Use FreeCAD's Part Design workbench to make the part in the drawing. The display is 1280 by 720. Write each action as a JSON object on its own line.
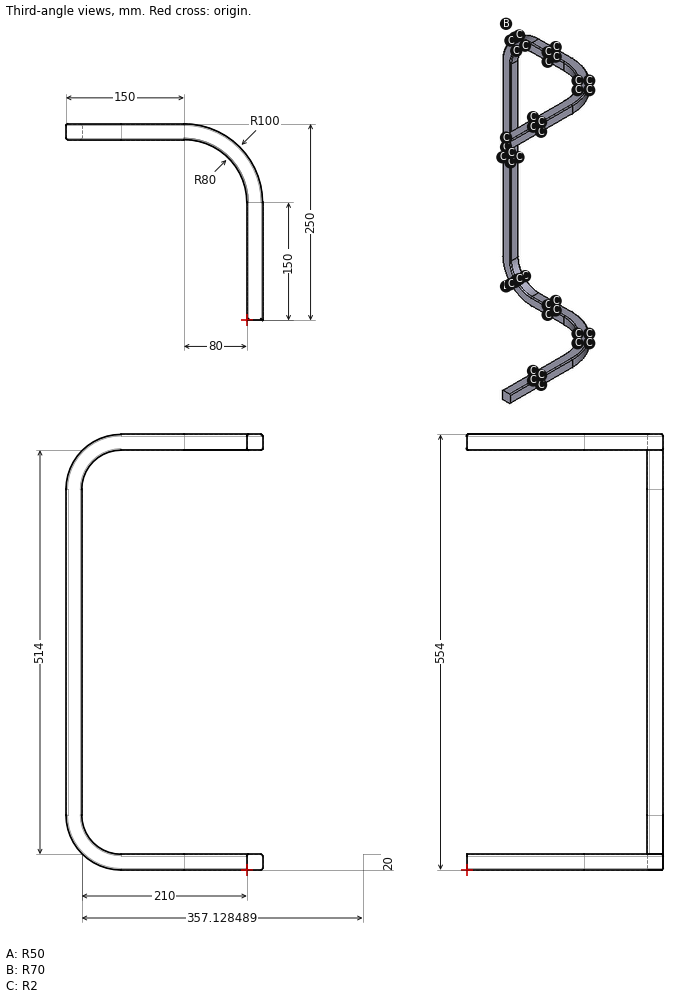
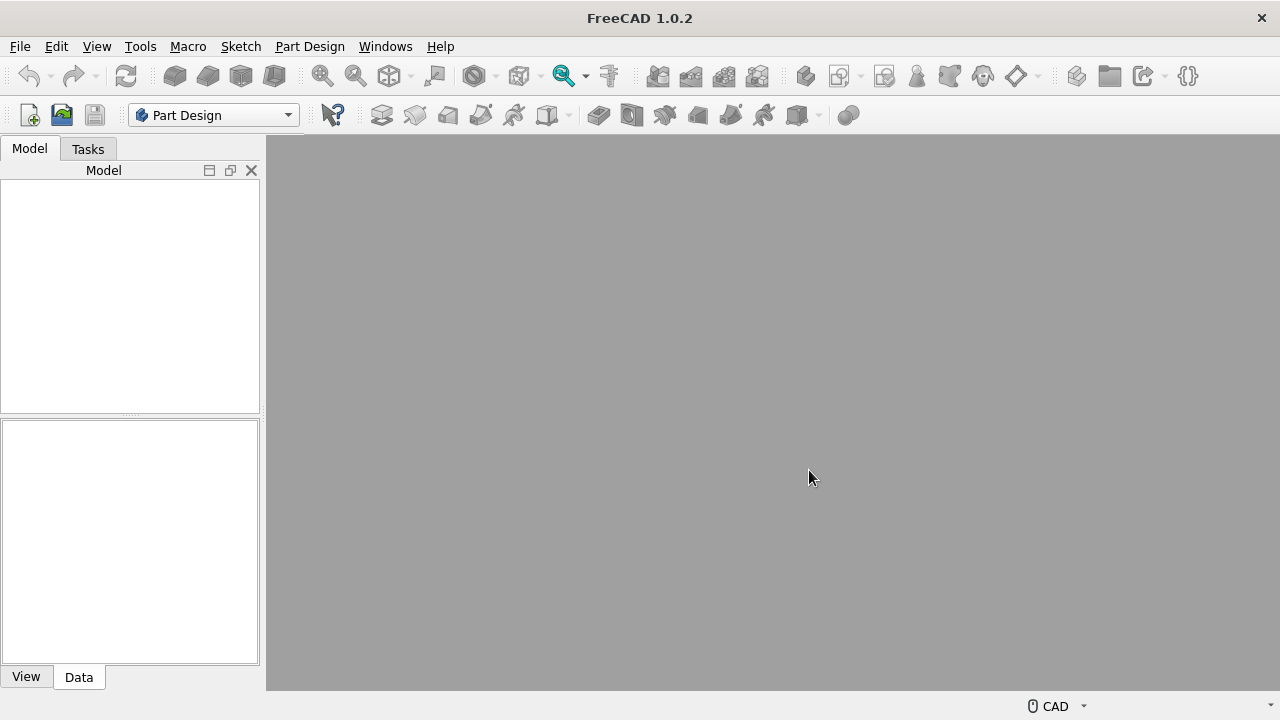
{"action": "left_click", "coordinate": [29, 116]}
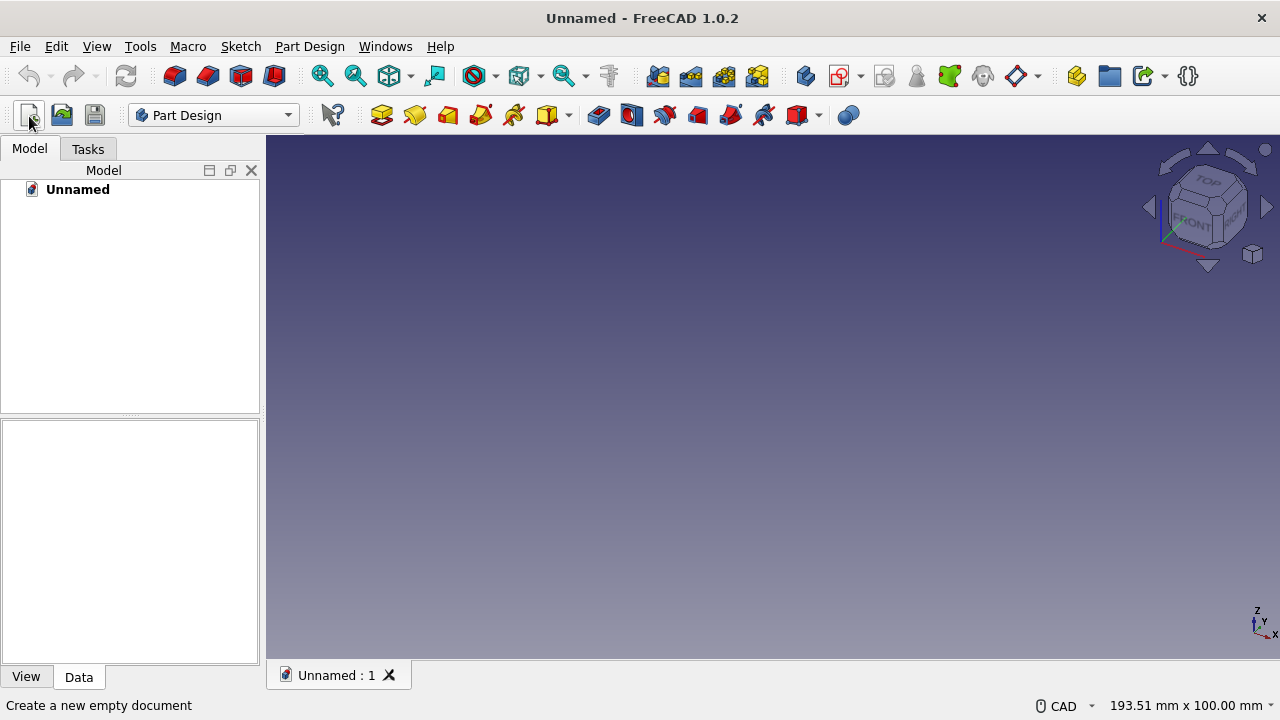
{"action": "left_click", "coordinate": [838, 76]}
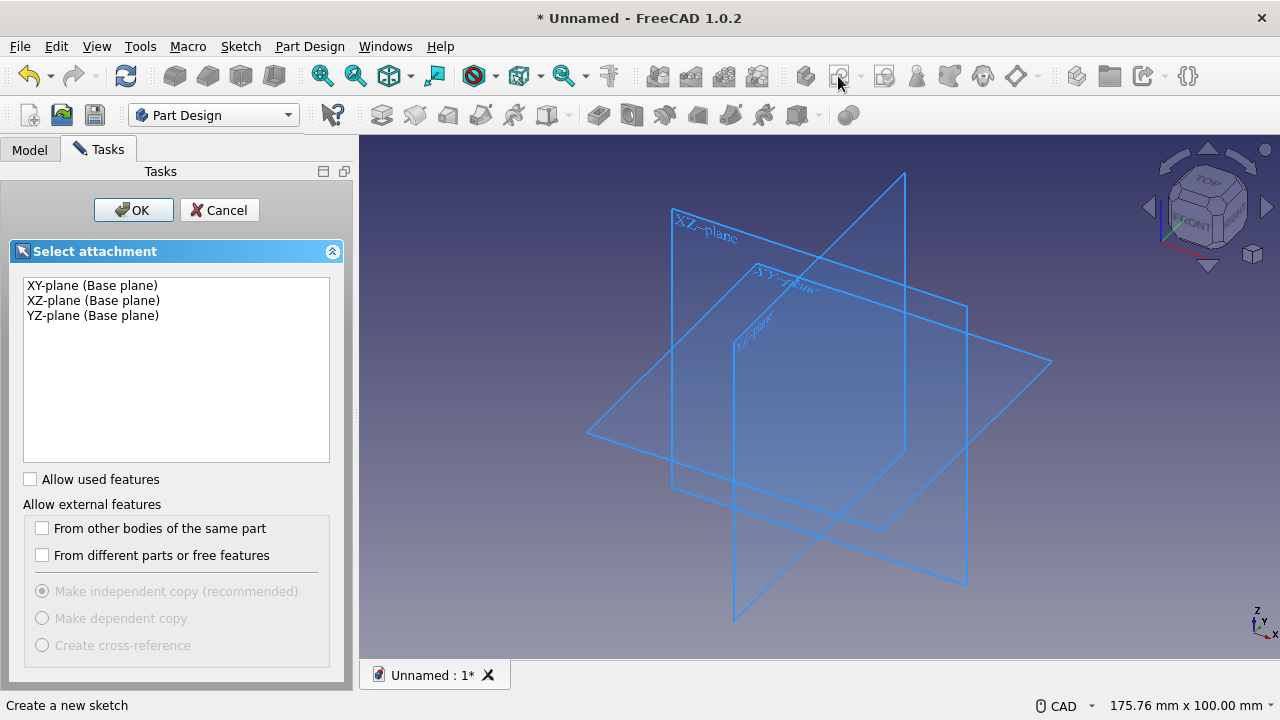
{"action": "left_click", "coordinate": [84, 286]}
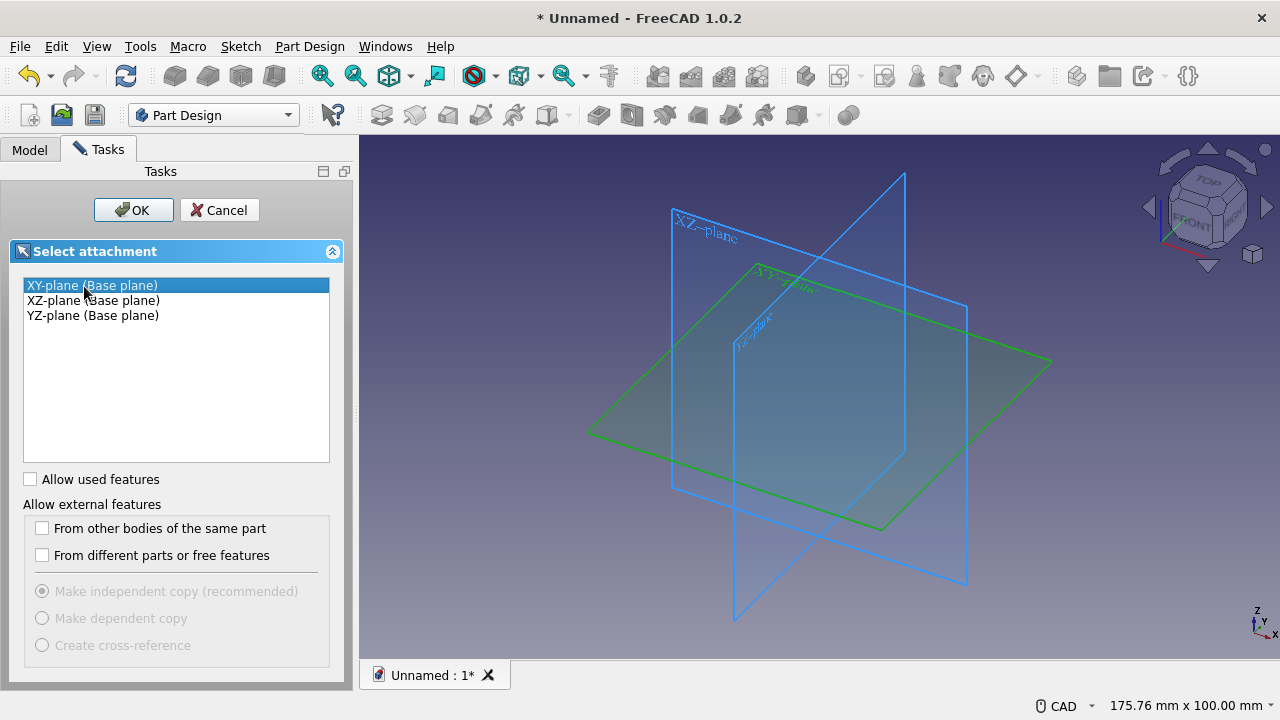
{"action": "left_click", "coordinate": [134, 210]}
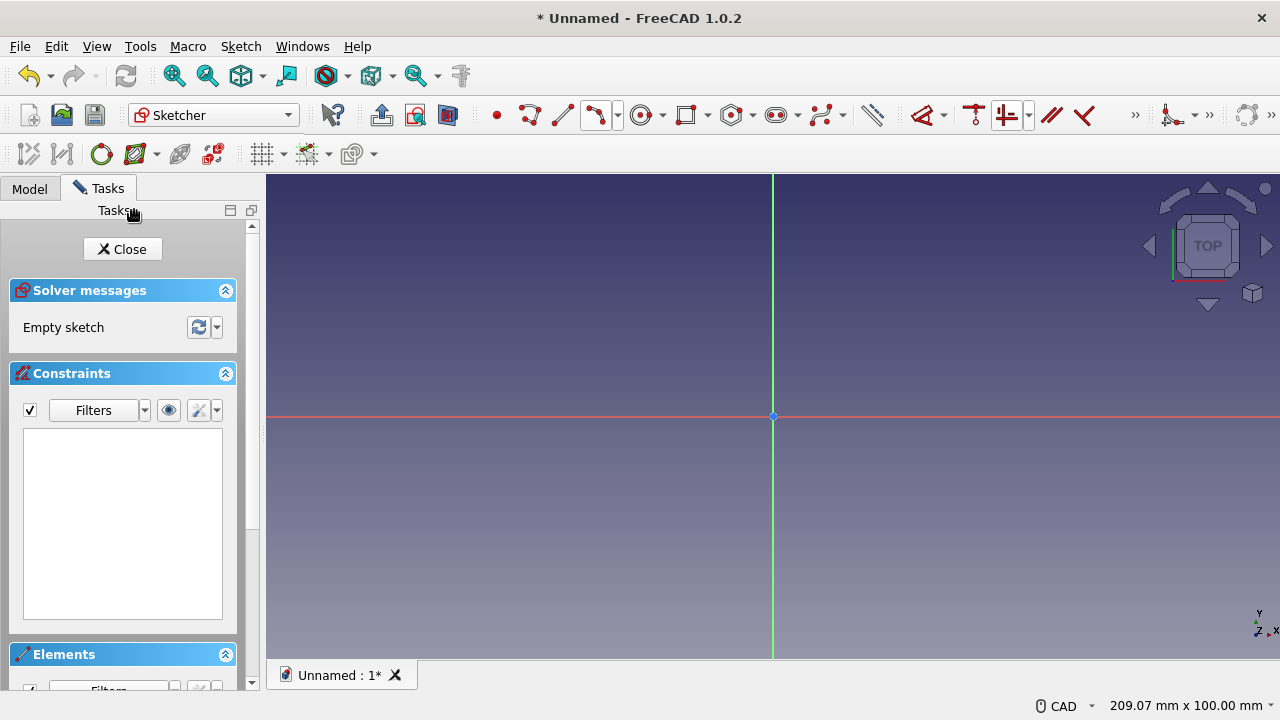
{"action": "scroll", "coordinate": [849, 615], "scroll_direction": "down", "scroll_amount": 7}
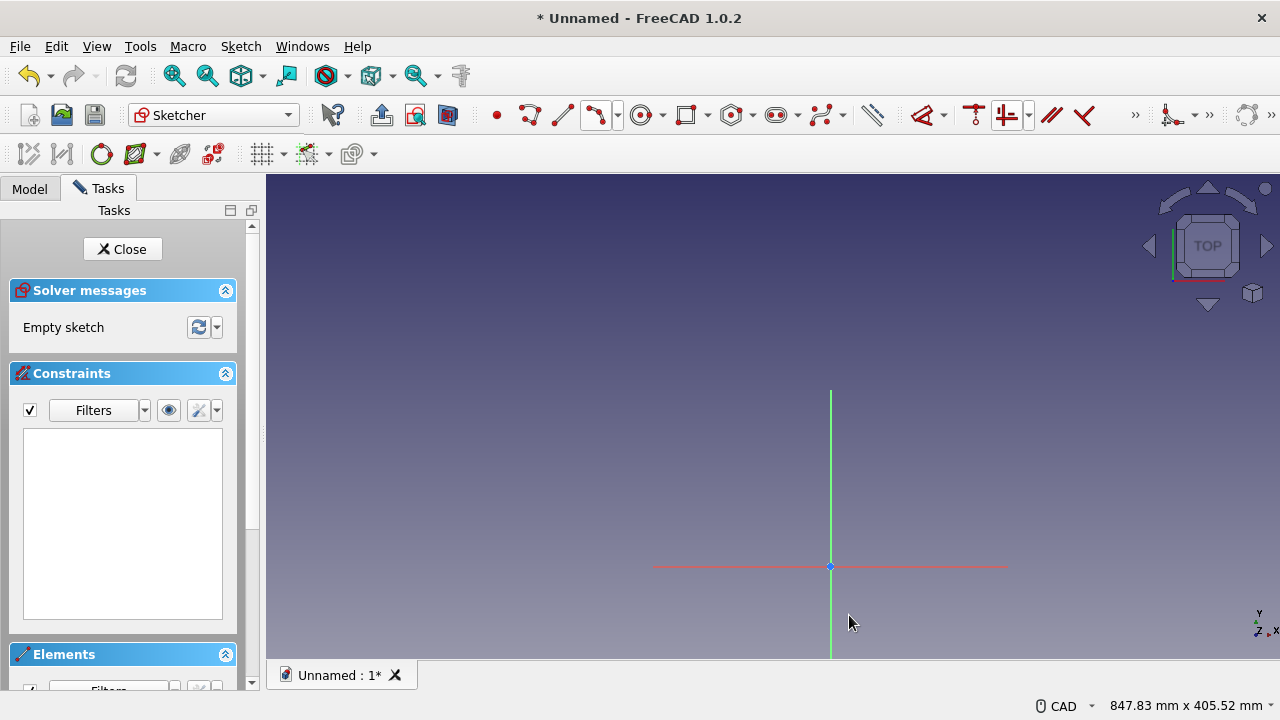
{"action": "left_click", "coordinate": [530, 116]}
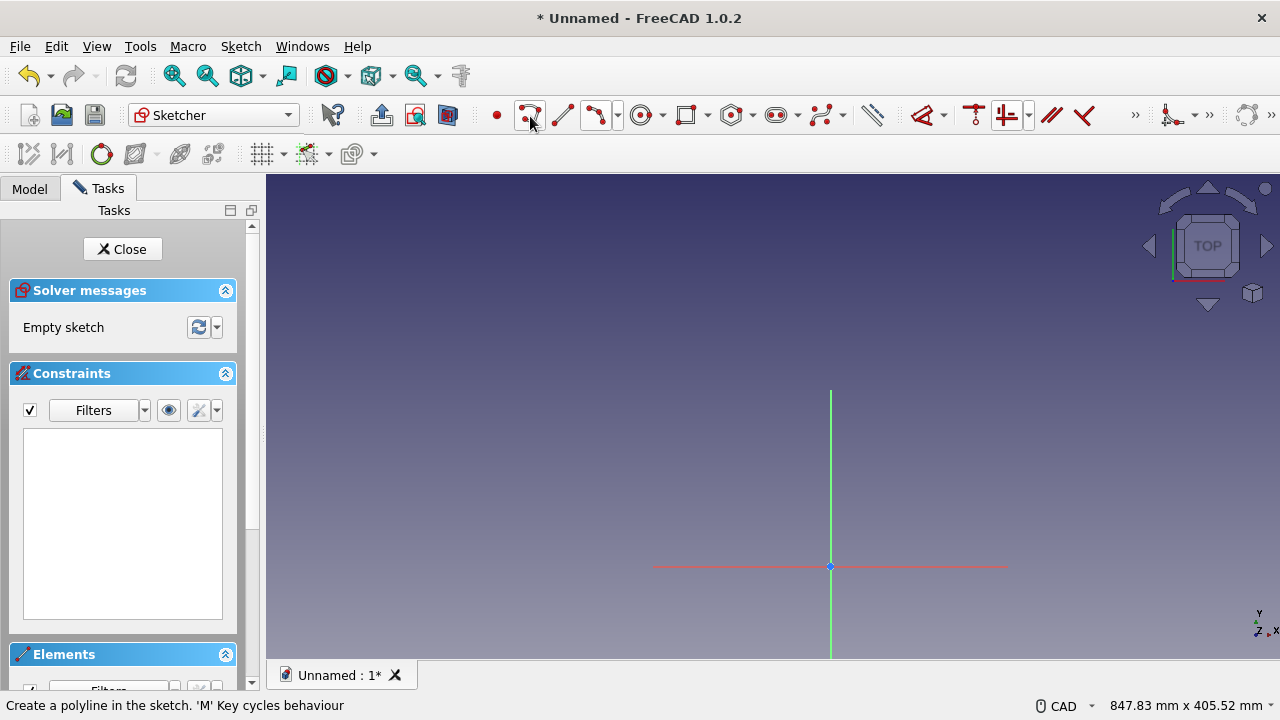
{"action": "left_click", "coordinate": [831, 387]}
{"action": "left_click", "coordinate": [831, 567]}
{"action": "left_click", "coordinate": [855, 558]}
{"action": "left_click", "coordinate": [855, 387]}
{"action": "right_click", "coordinate": [855, 387]}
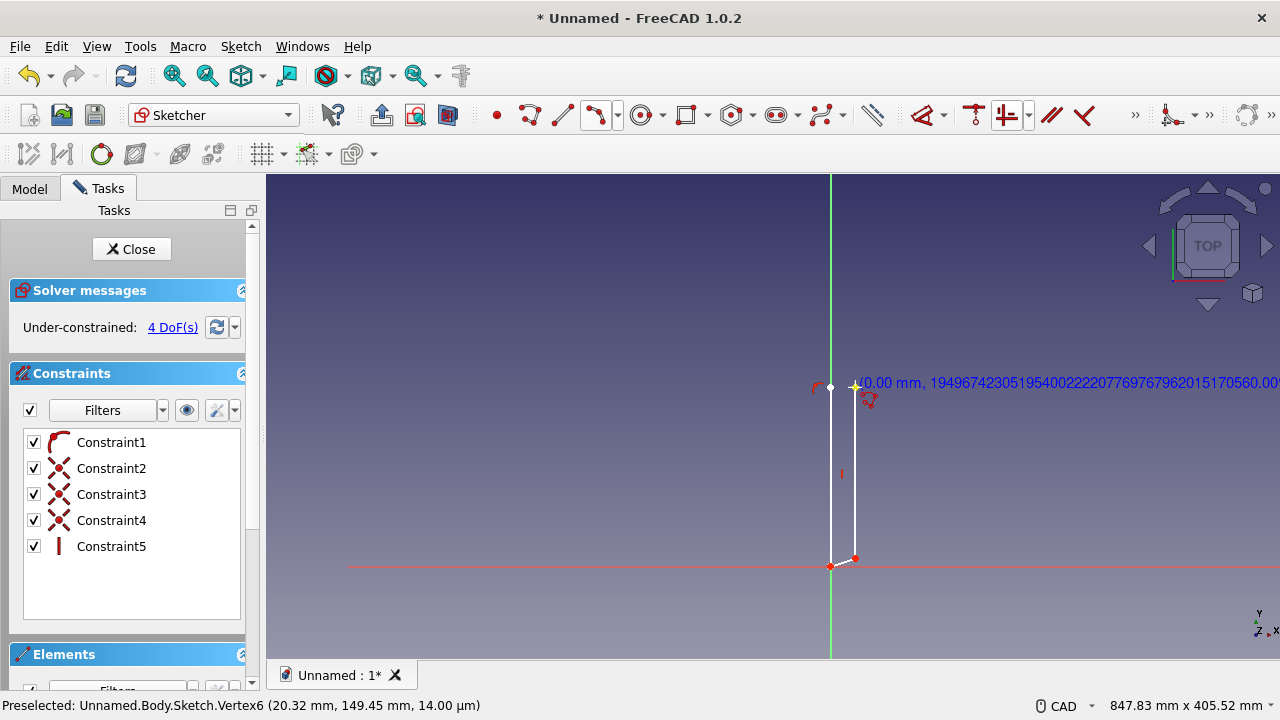
{"action": "left_click", "coordinate": [735, 268]}
{"action": "left_click", "coordinate": [556, 268]}
{"action": "left_click", "coordinate": [556, 292]}
{"action": "left_click", "coordinate": [735, 292]}
{"action": "right_click", "coordinate": [735, 292]}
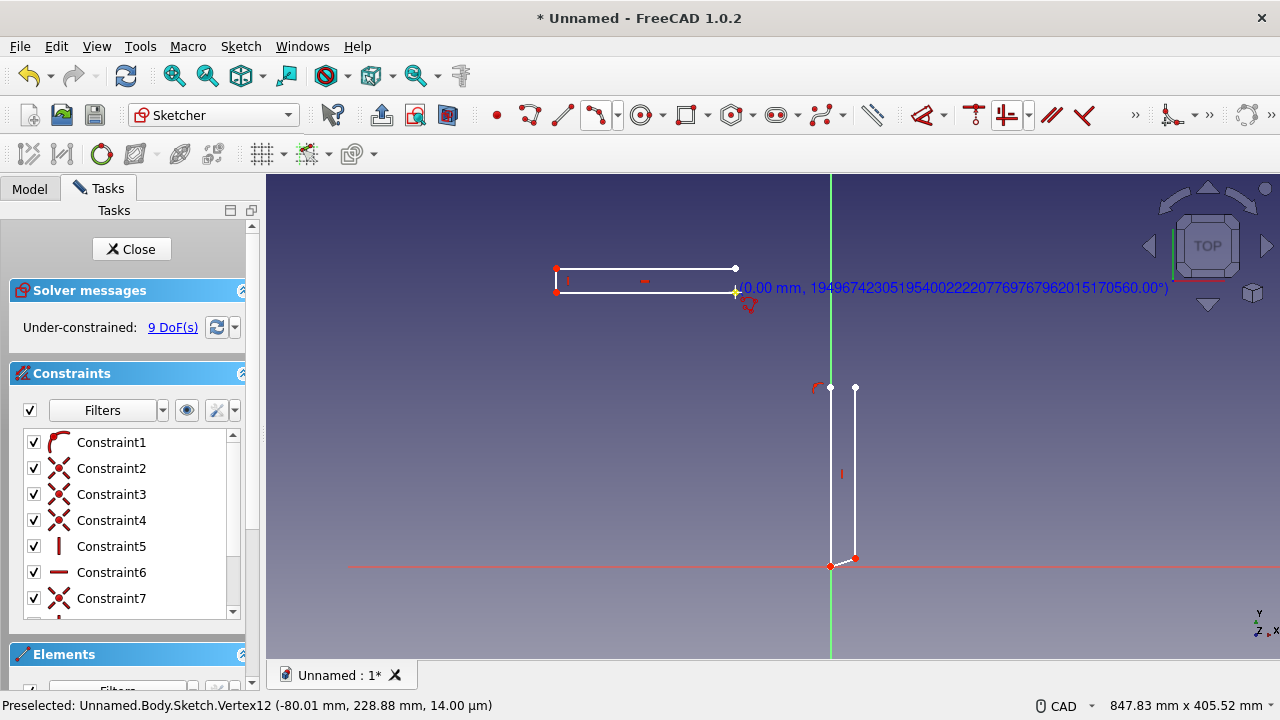
{"action": "left_click", "coordinate": [596, 116]}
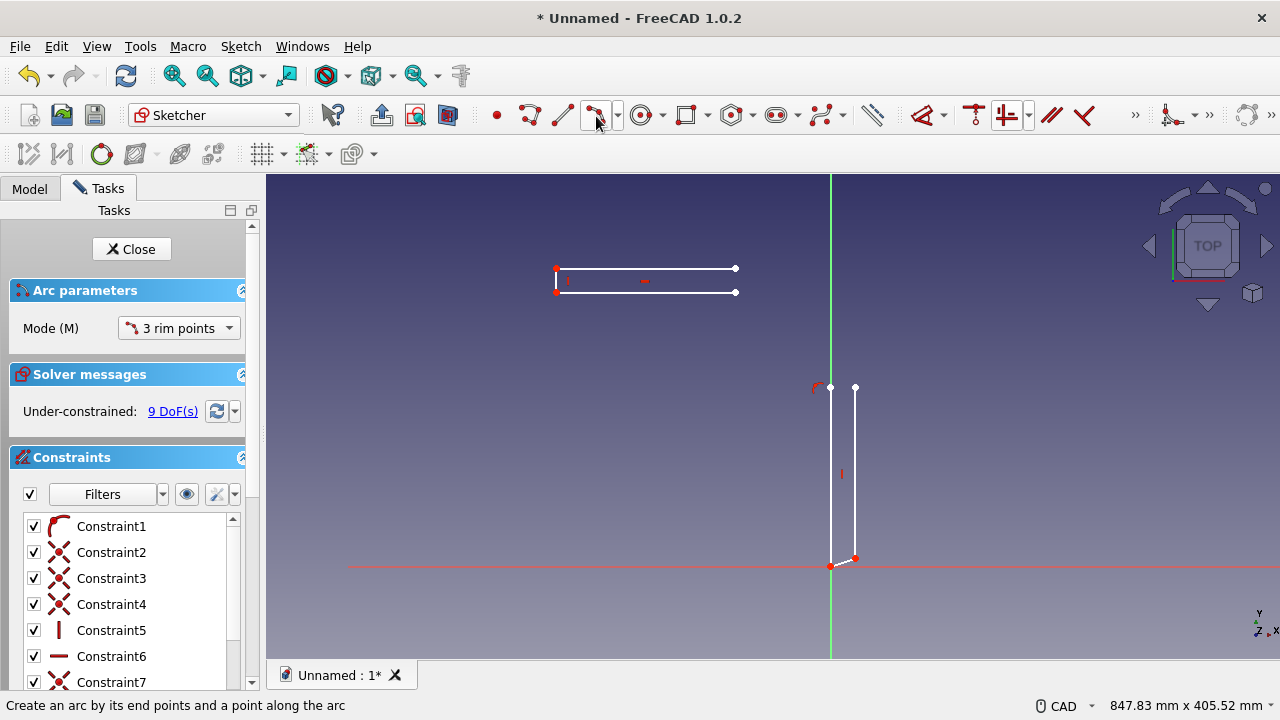
{"action": "left_click", "coordinate": [855, 388]}
{"action": "left_click", "coordinate": [735, 269]}
{"action": "left_click", "coordinate": [805, 291]}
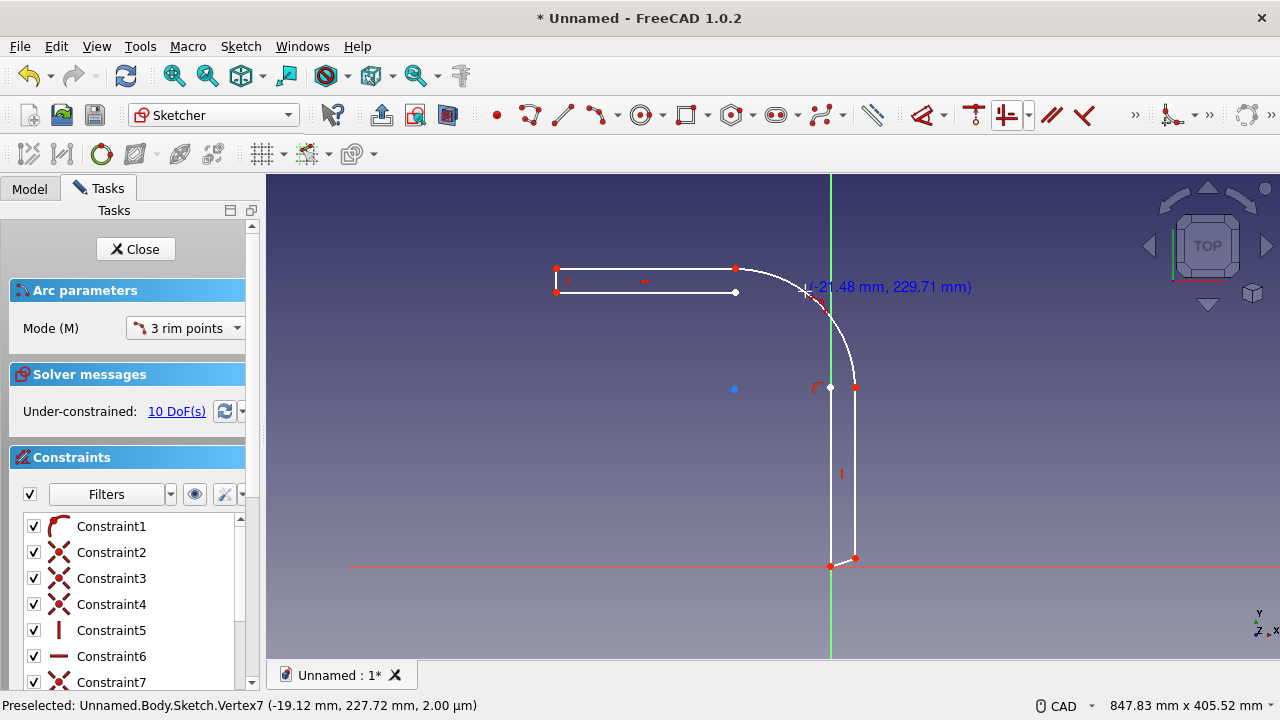
{"action": "left_click", "coordinate": [735, 293]}
{"action": "left_click", "coordinate": [831, 388]}
{"action": "left_click", "coordinate": [803, 320]}
{"action": "key", "text": "Escape"}